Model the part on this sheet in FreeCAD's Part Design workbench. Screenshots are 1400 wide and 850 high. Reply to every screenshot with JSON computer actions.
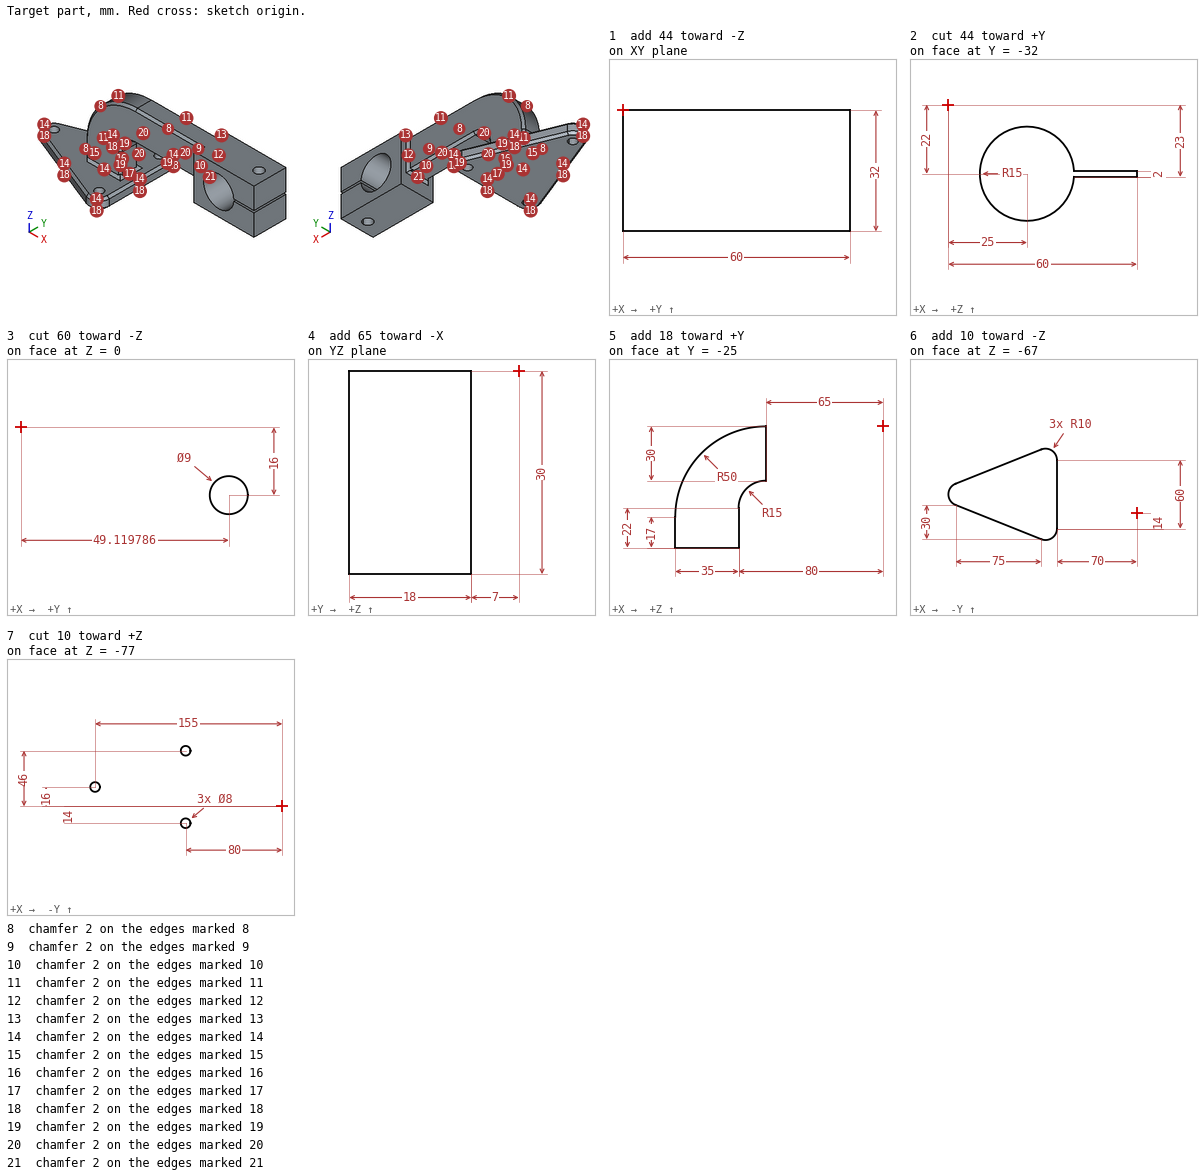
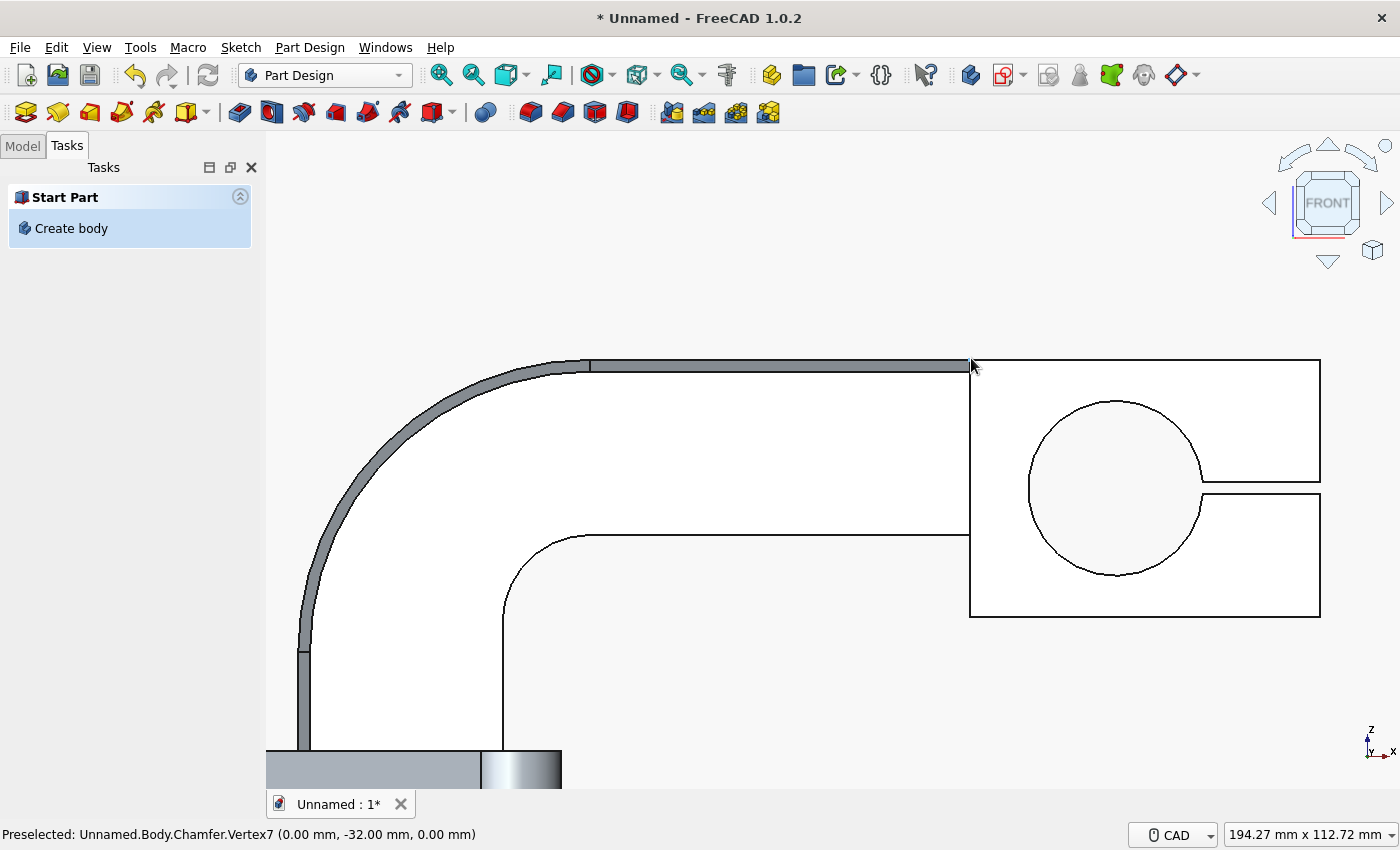
{"action": "left_click", "coordinate": [442, 76]}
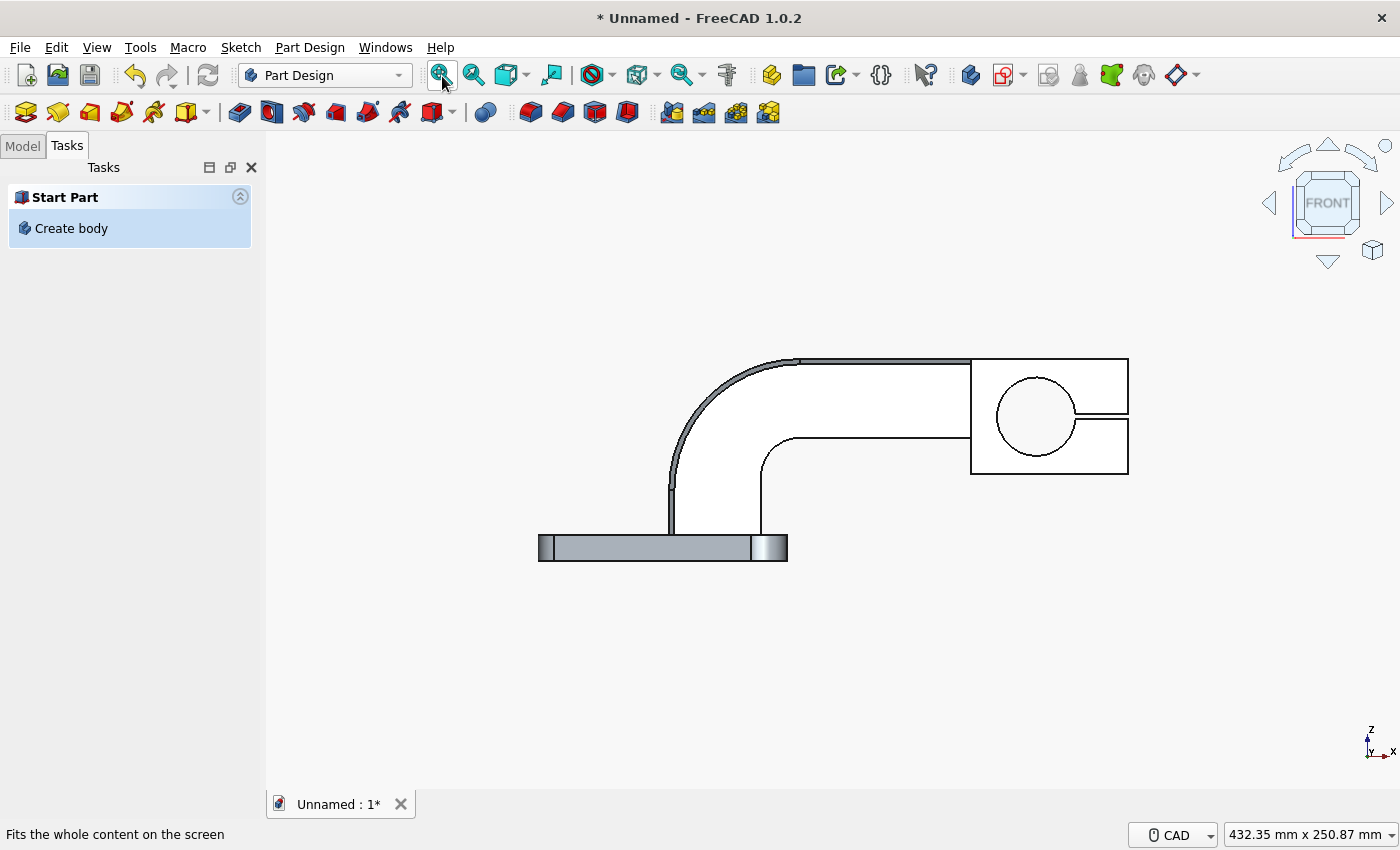
{"action": "key", "text": "0"}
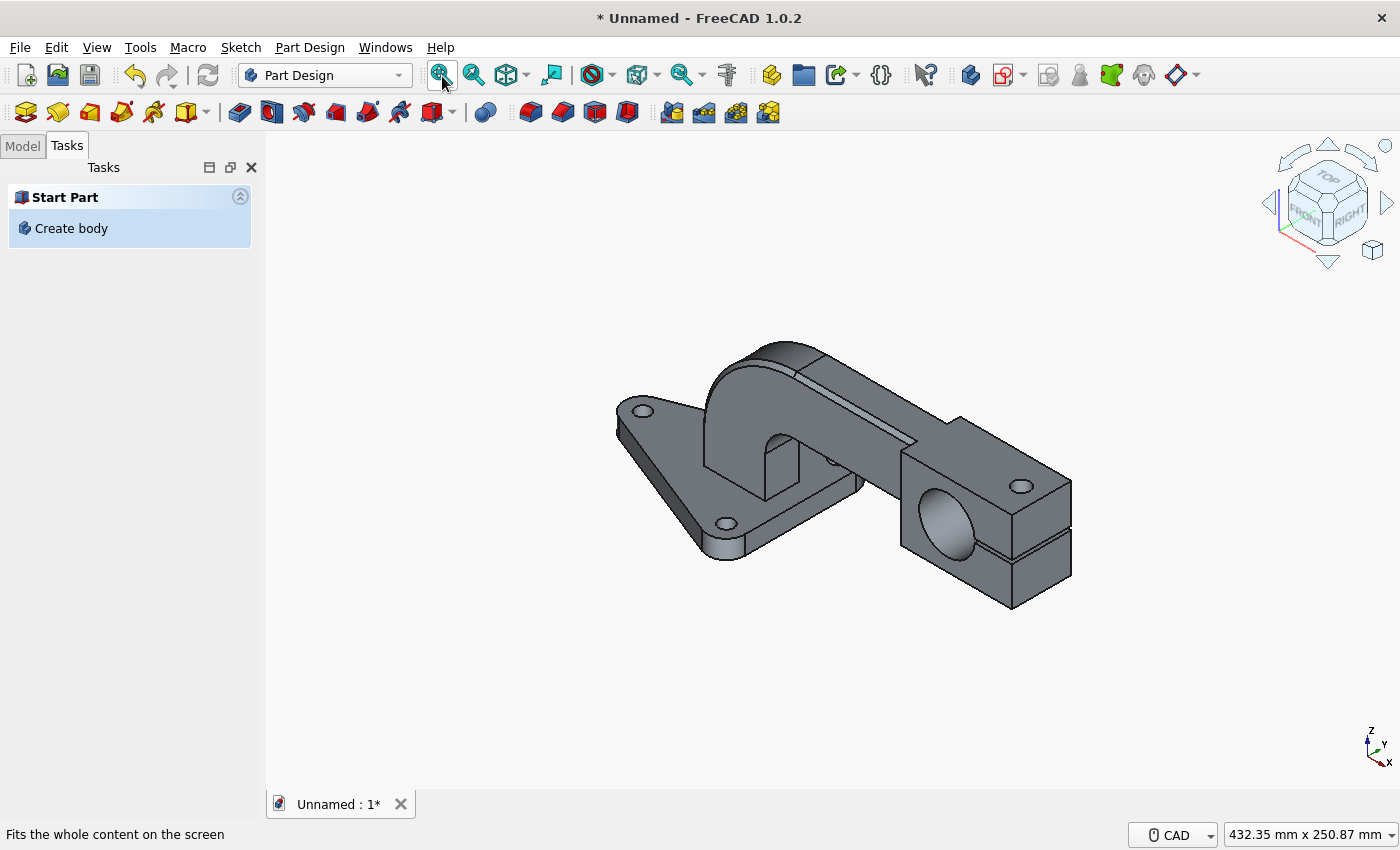
{"action": "scroll", "coordinate": [907, 446], "scroll_direction": "up", "scroll_amount": 4}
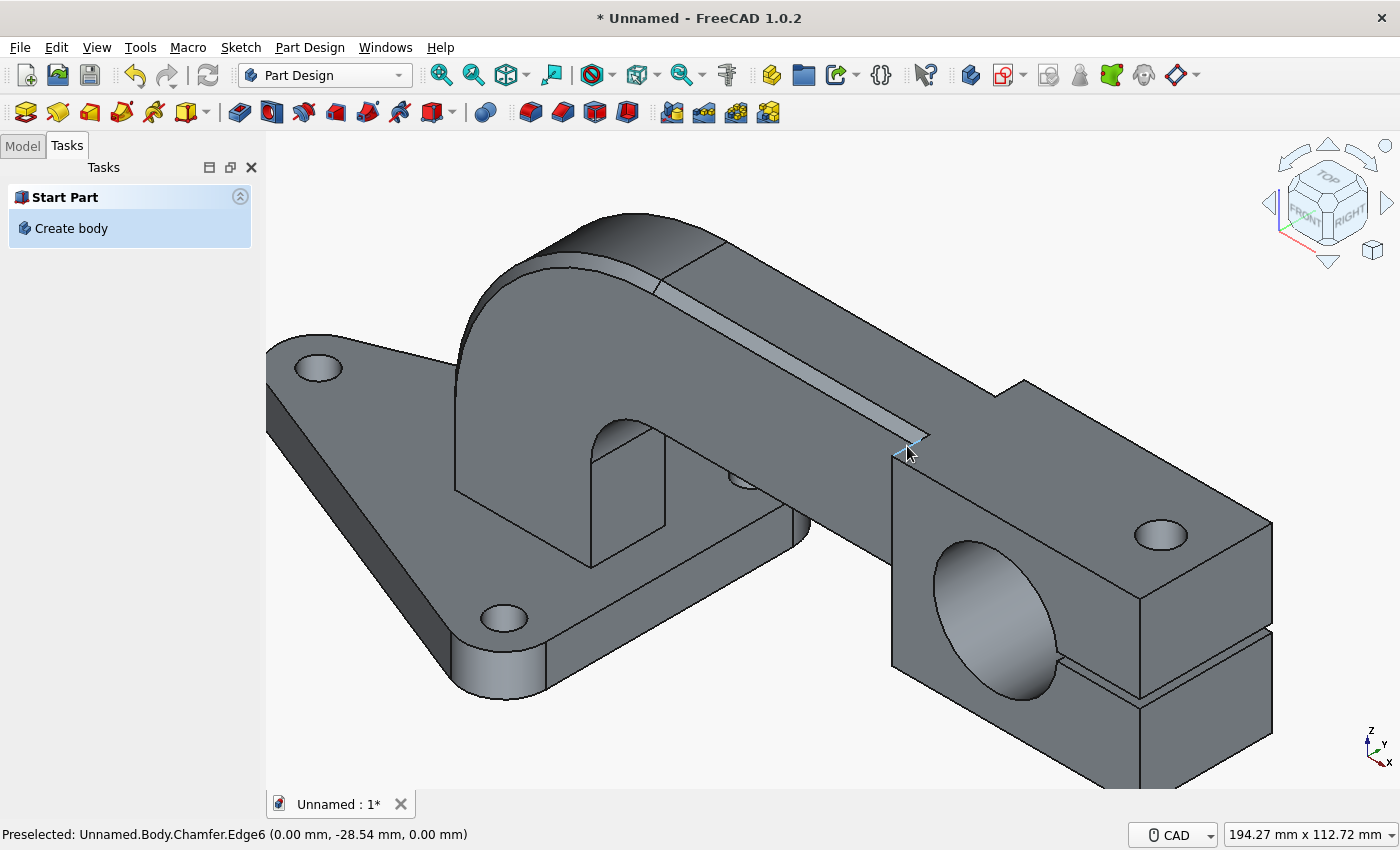
{"action": "left_click", "coordinate": [442, 76]}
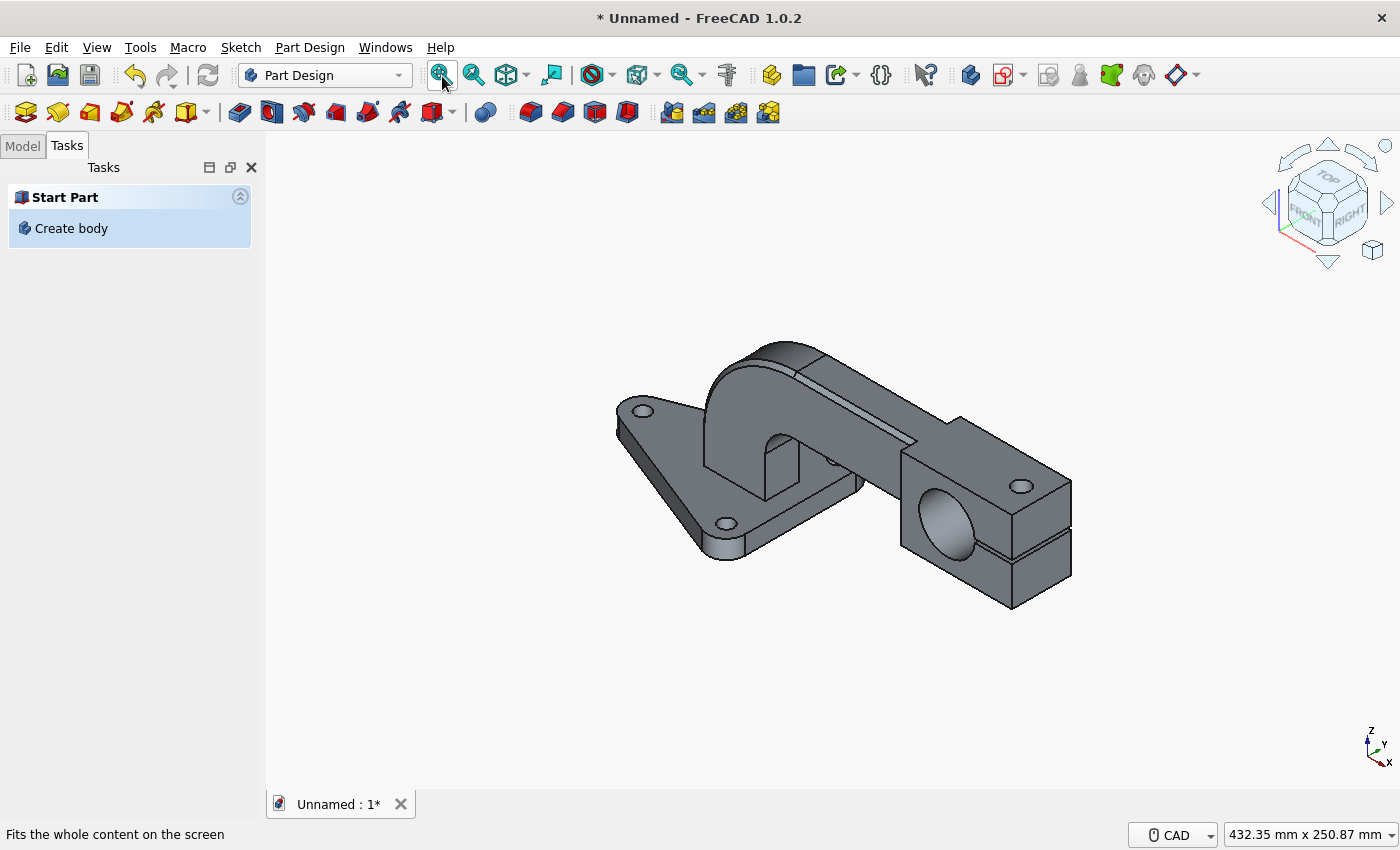
{"action": "key", "text": "2"}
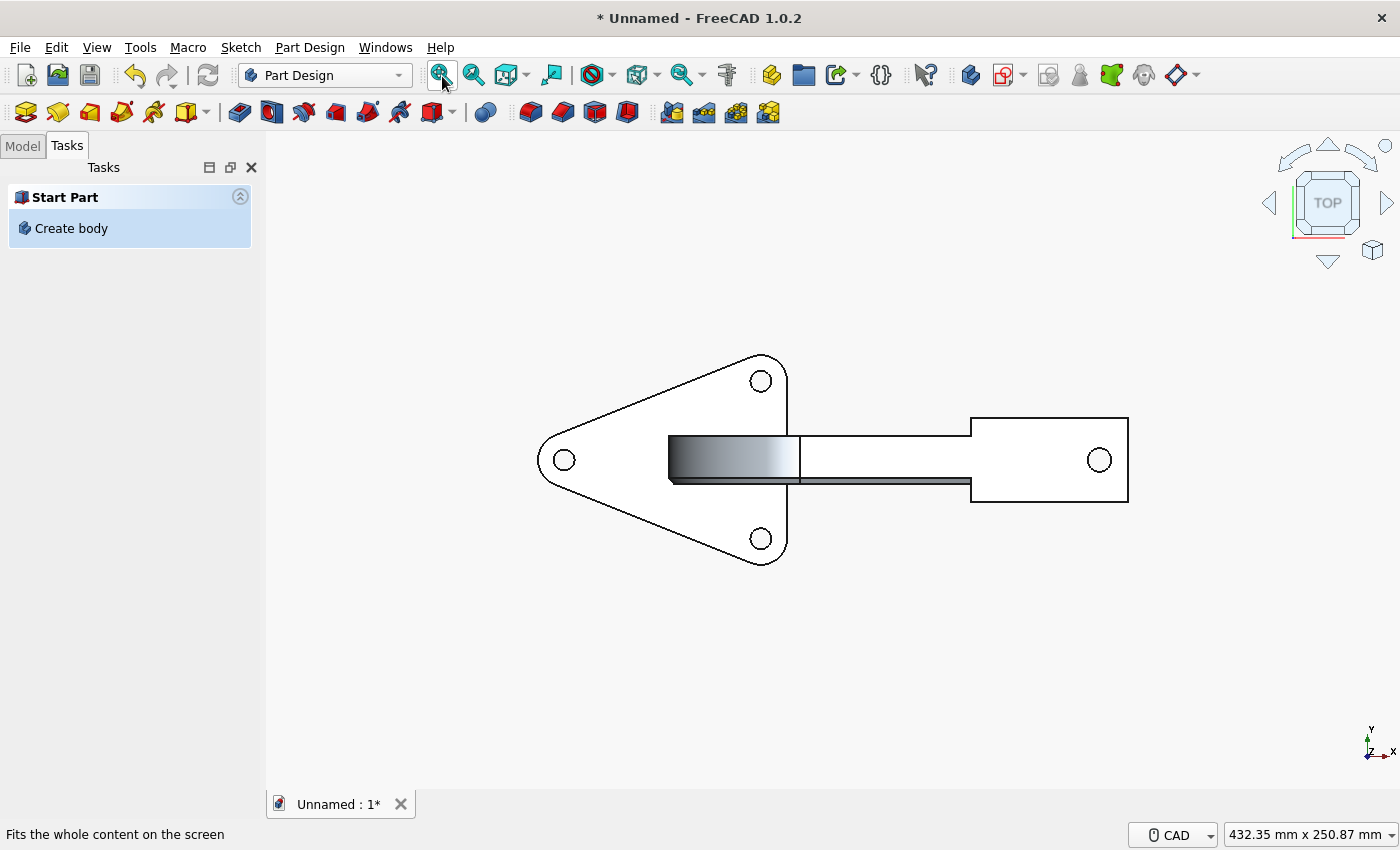
{"action": "left_click", "coordinate": [971, 492]}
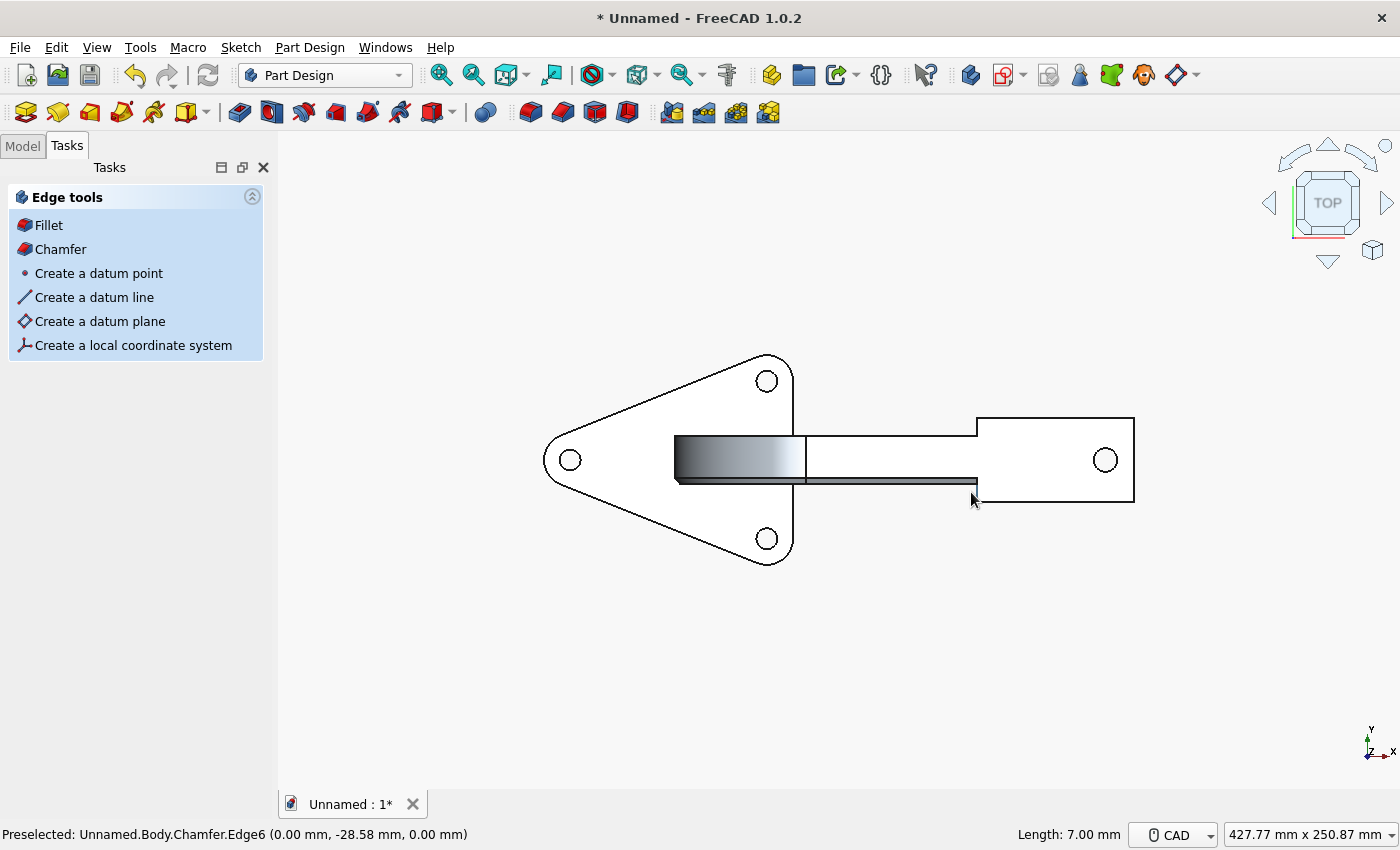
{"action": "left_click", "coordinate": [564, 112]}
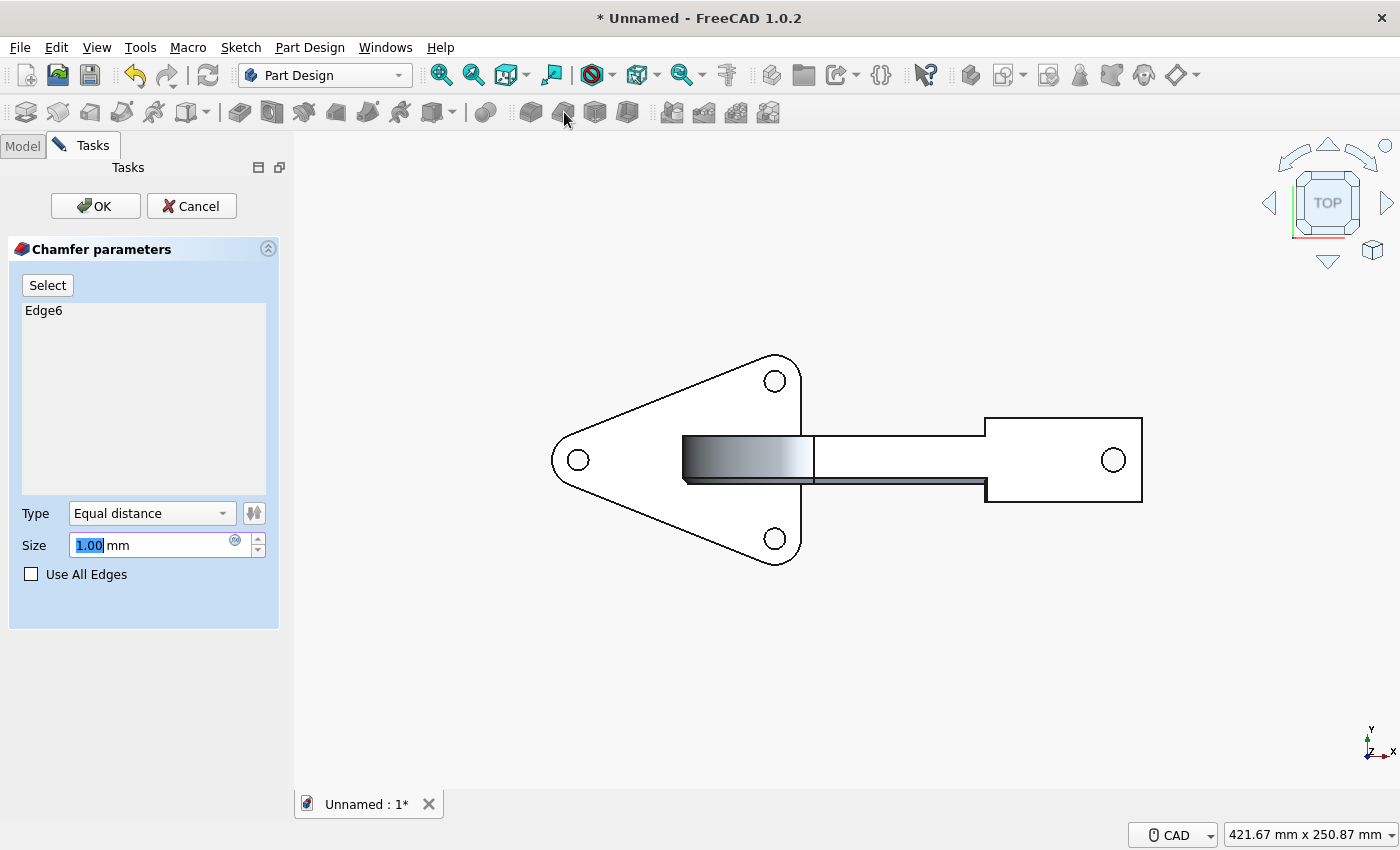
{"action": "type", "text": "2"}
{"action": "key", "text": "Tab"}